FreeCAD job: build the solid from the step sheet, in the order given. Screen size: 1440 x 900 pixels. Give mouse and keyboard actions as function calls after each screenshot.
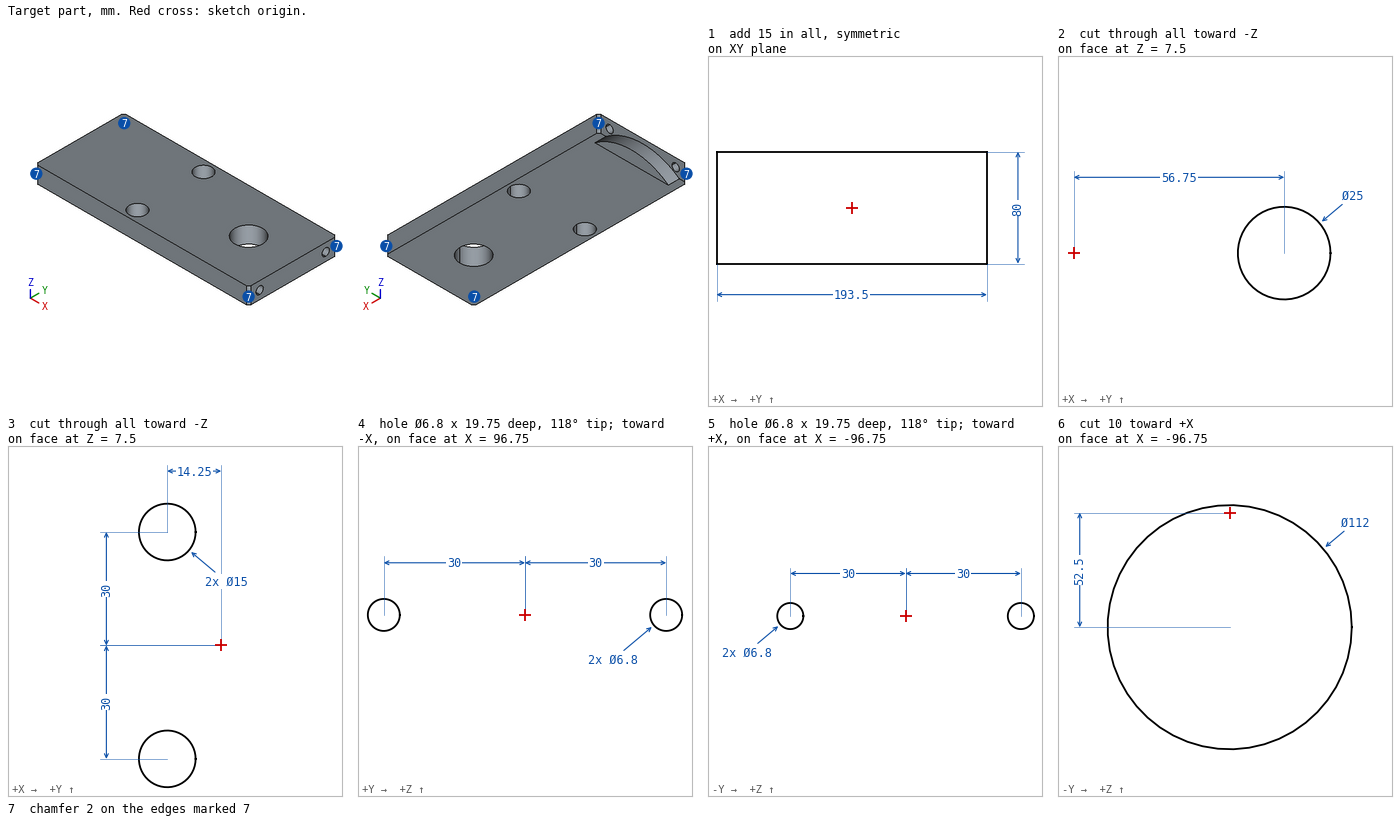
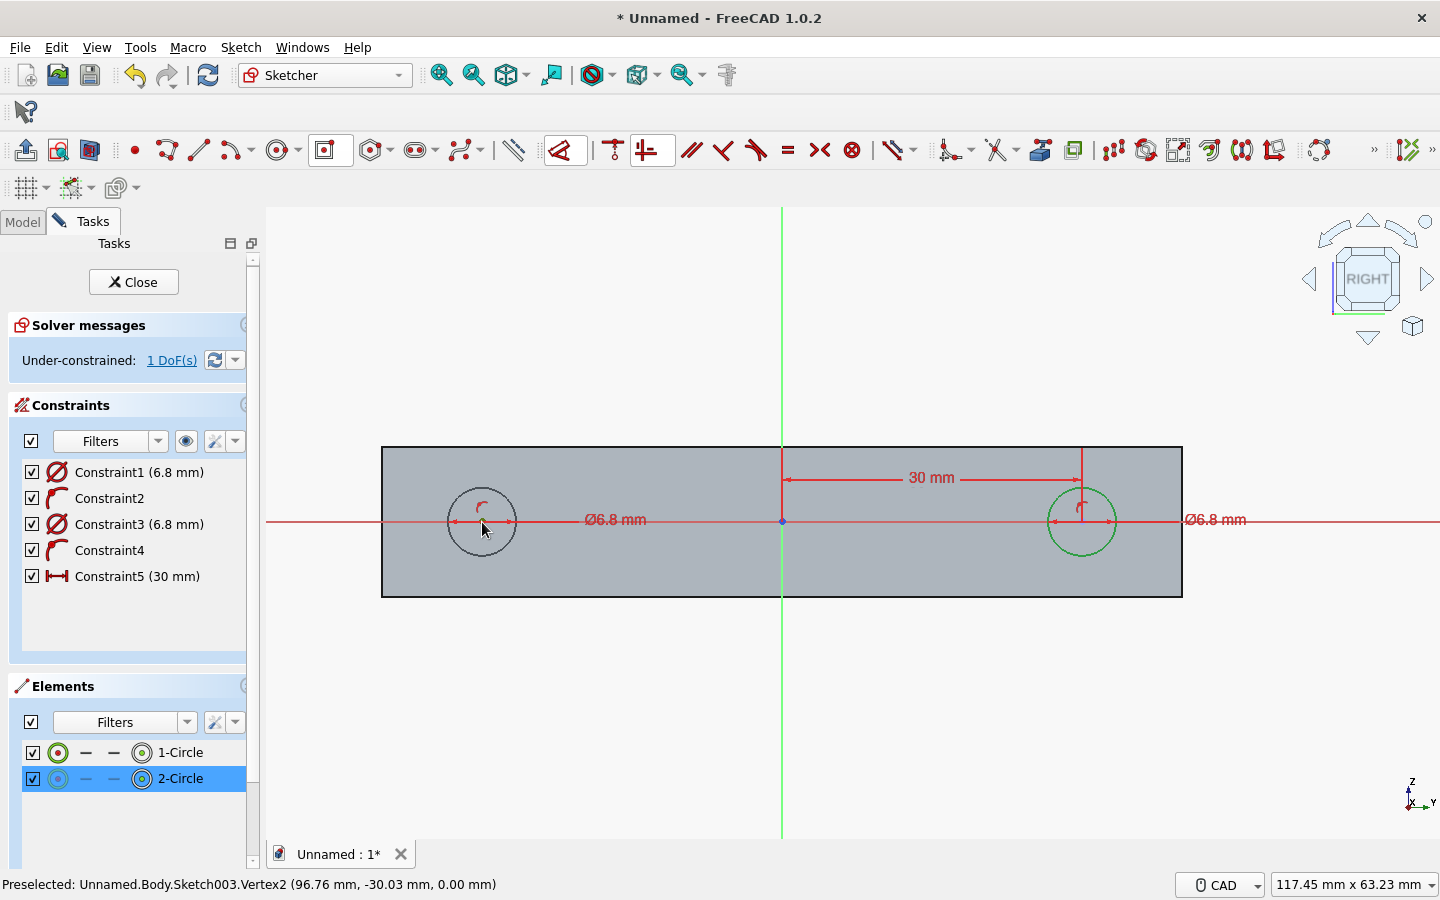
key(l)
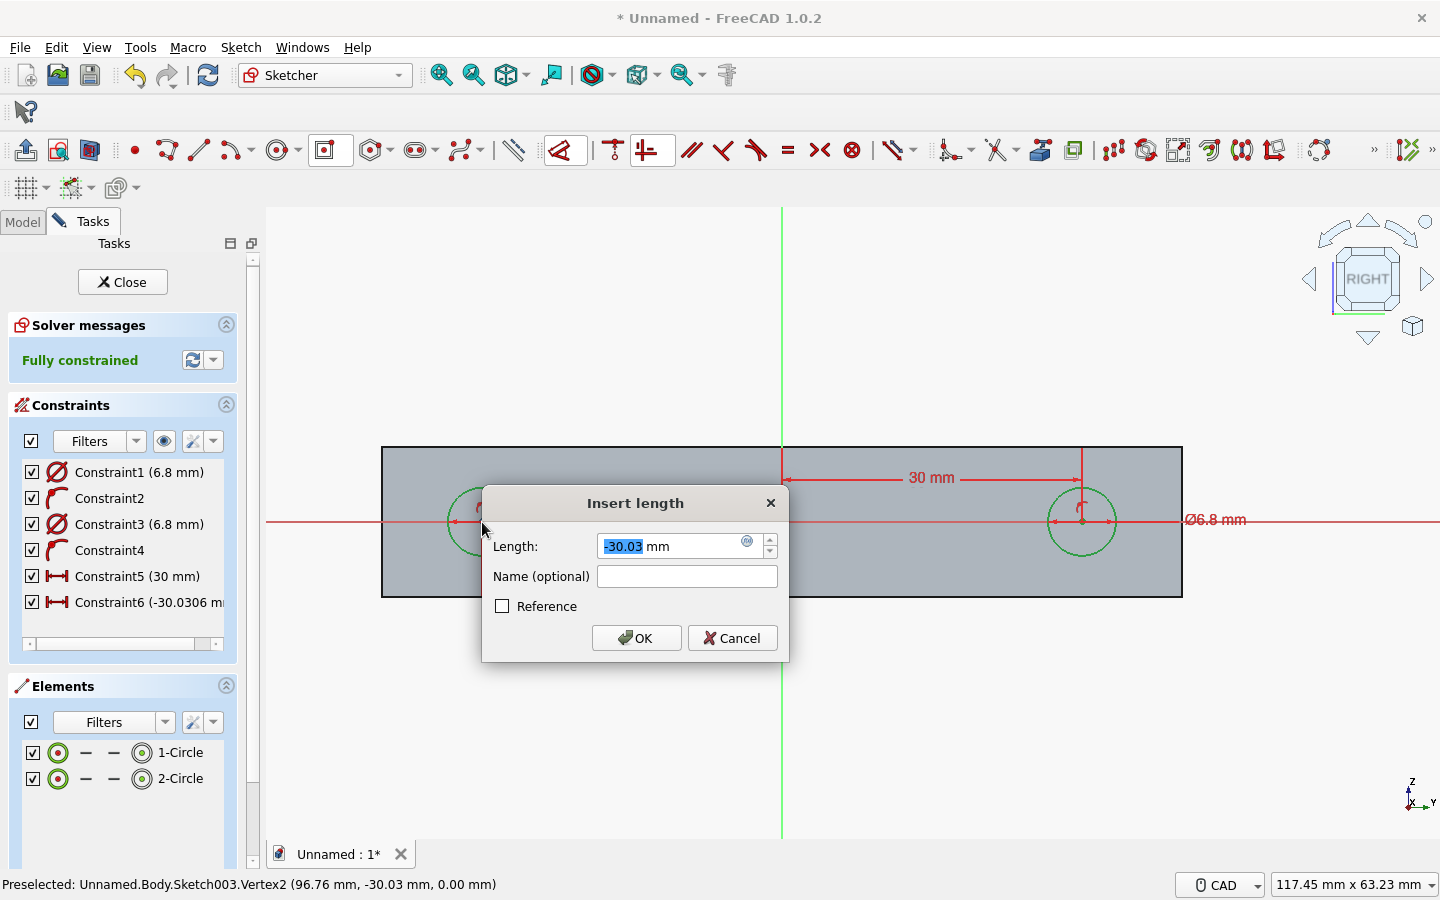
text(-30)
key(Return)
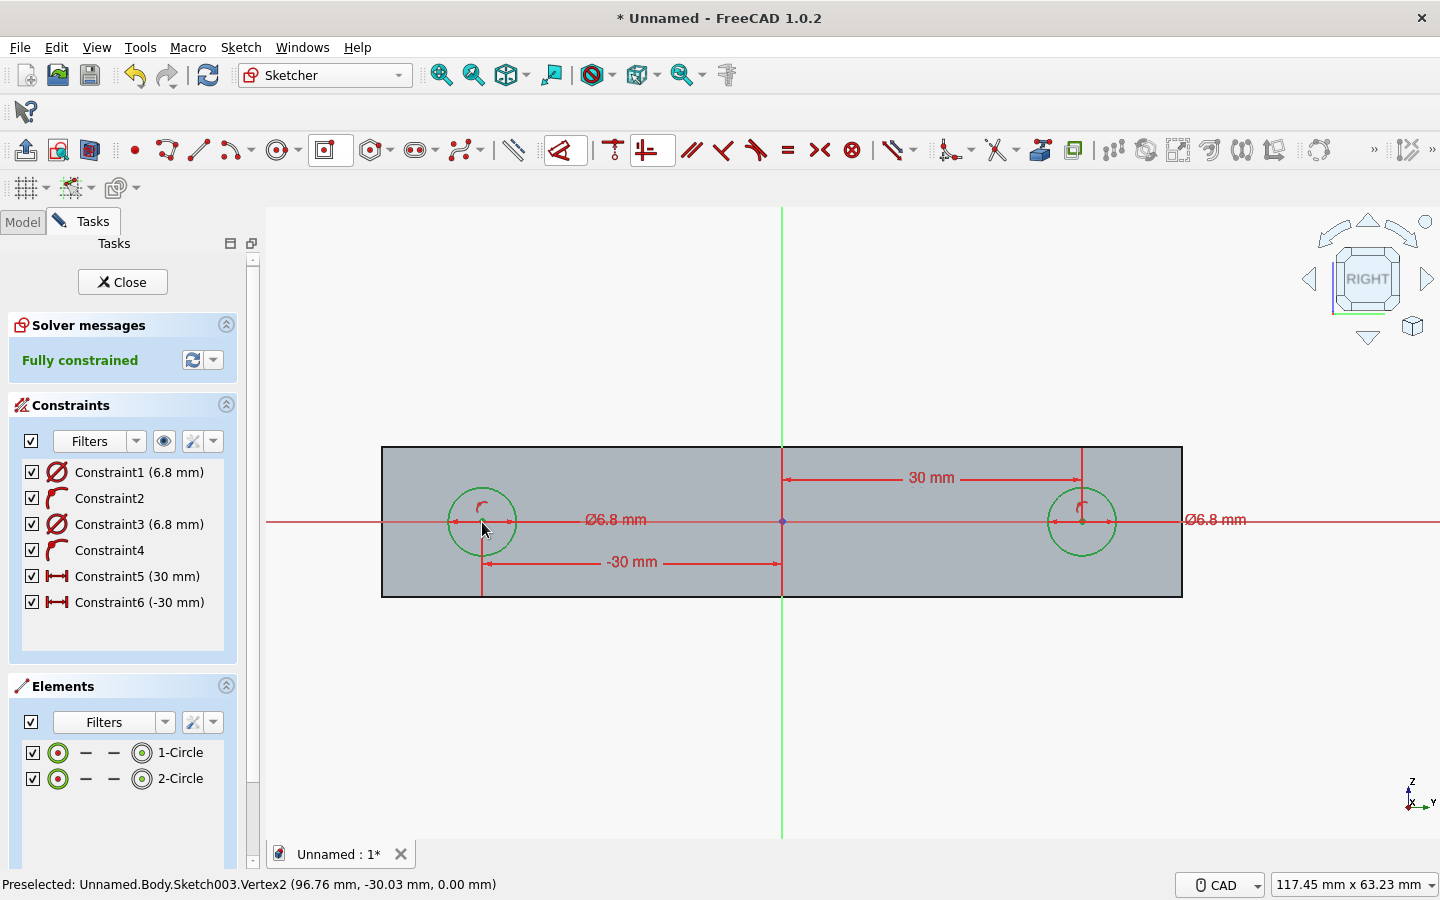
click(123, 282)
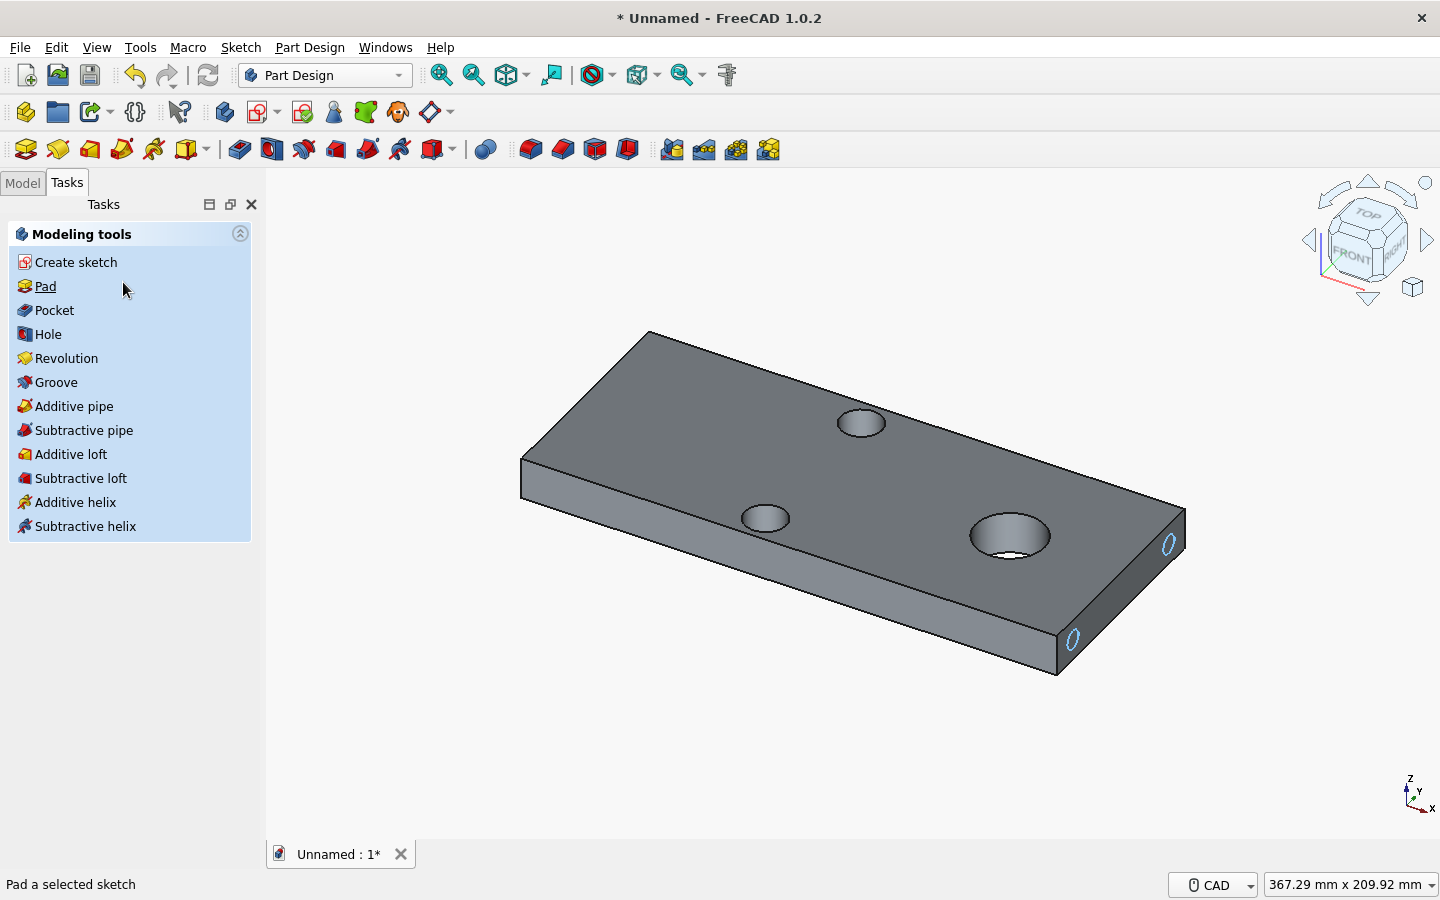
click(272, 150)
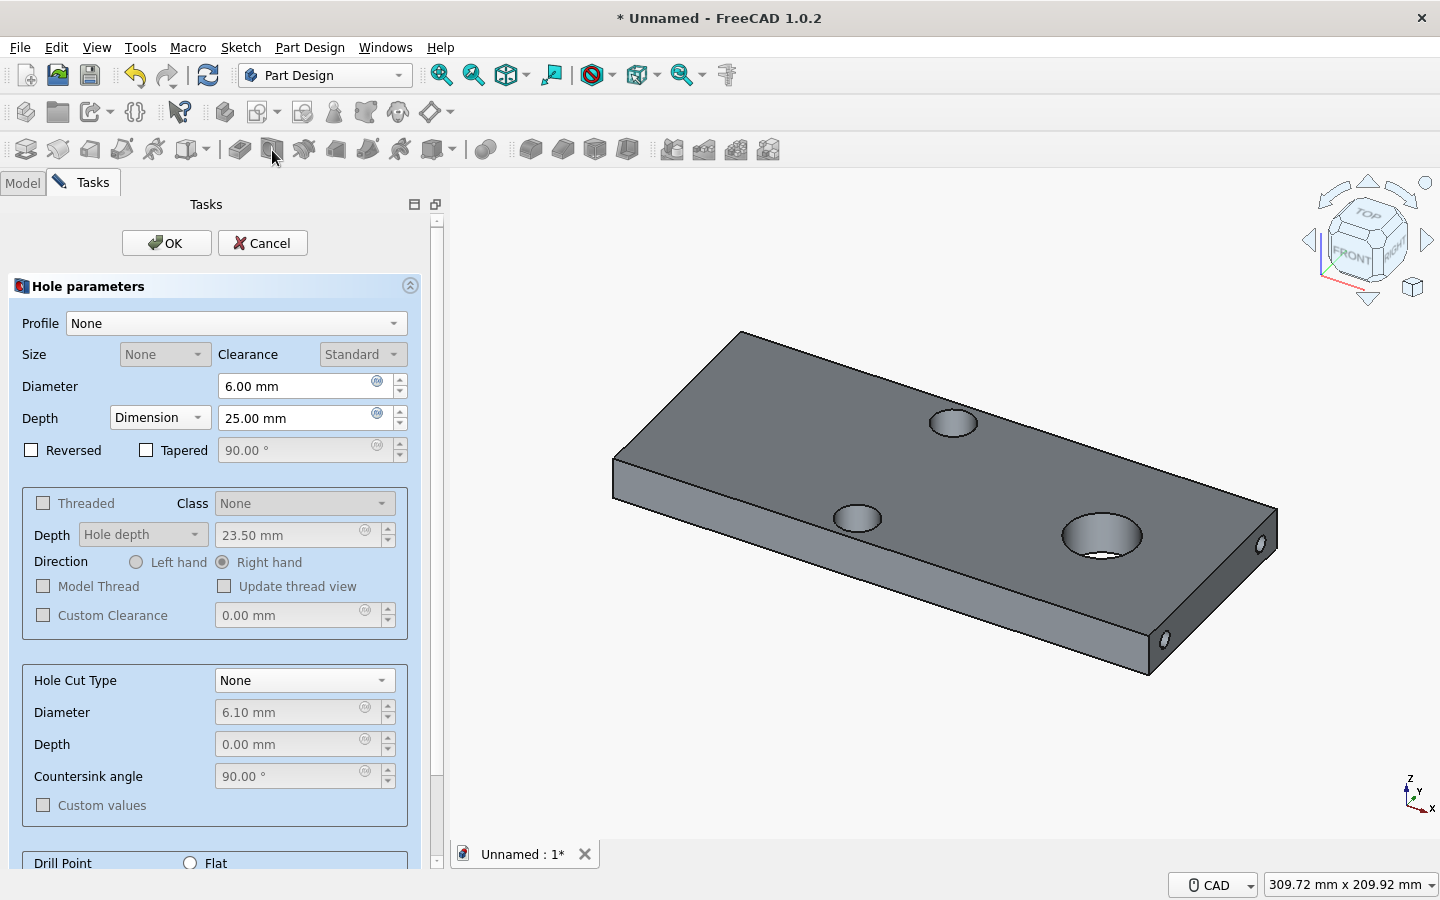
triple_click(305, 386)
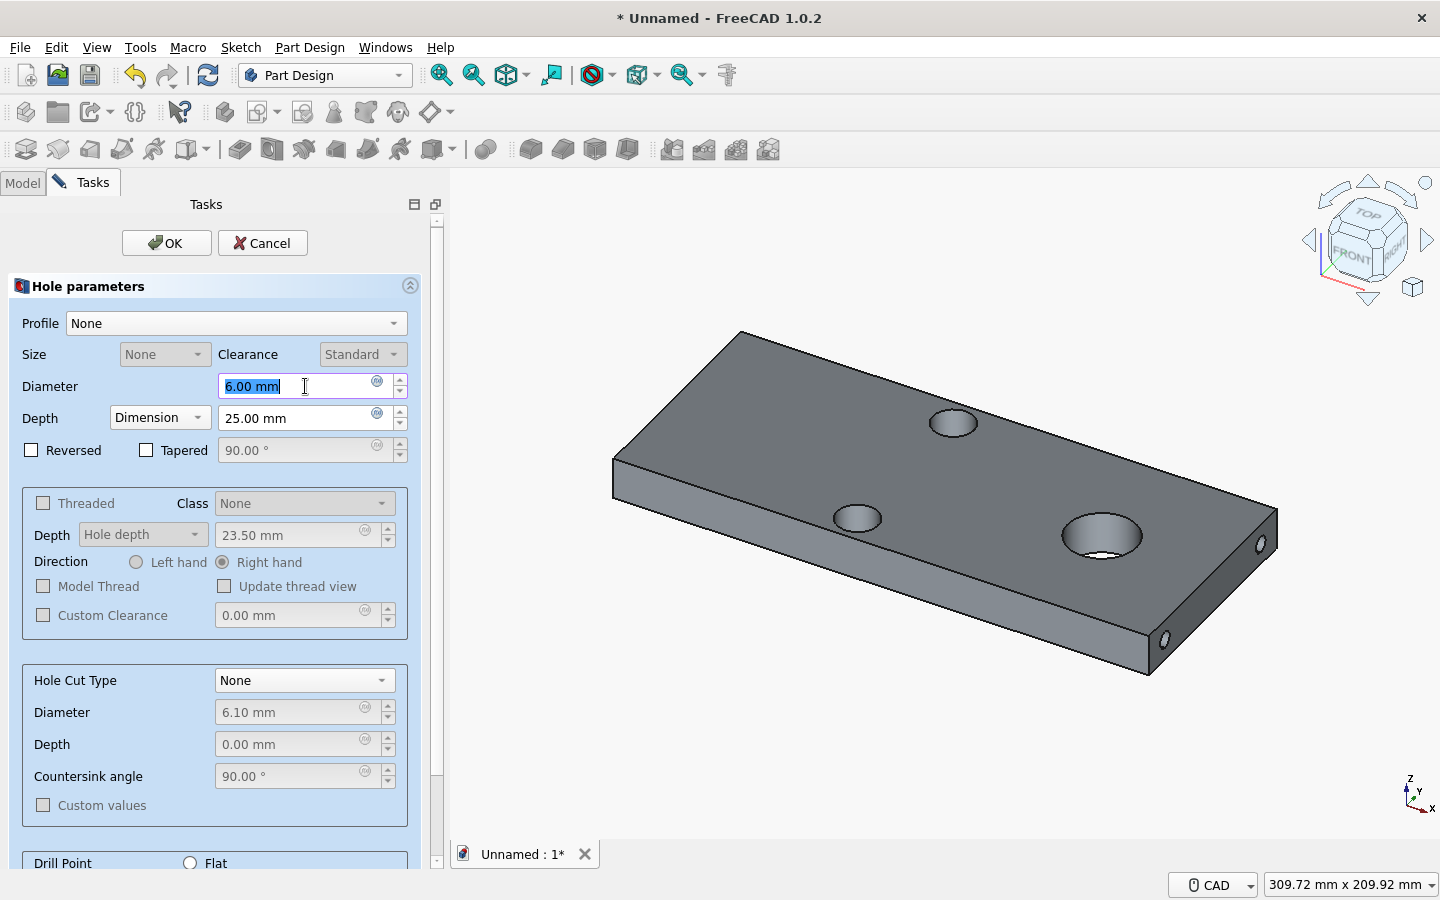
text(6.8)
key(Tab)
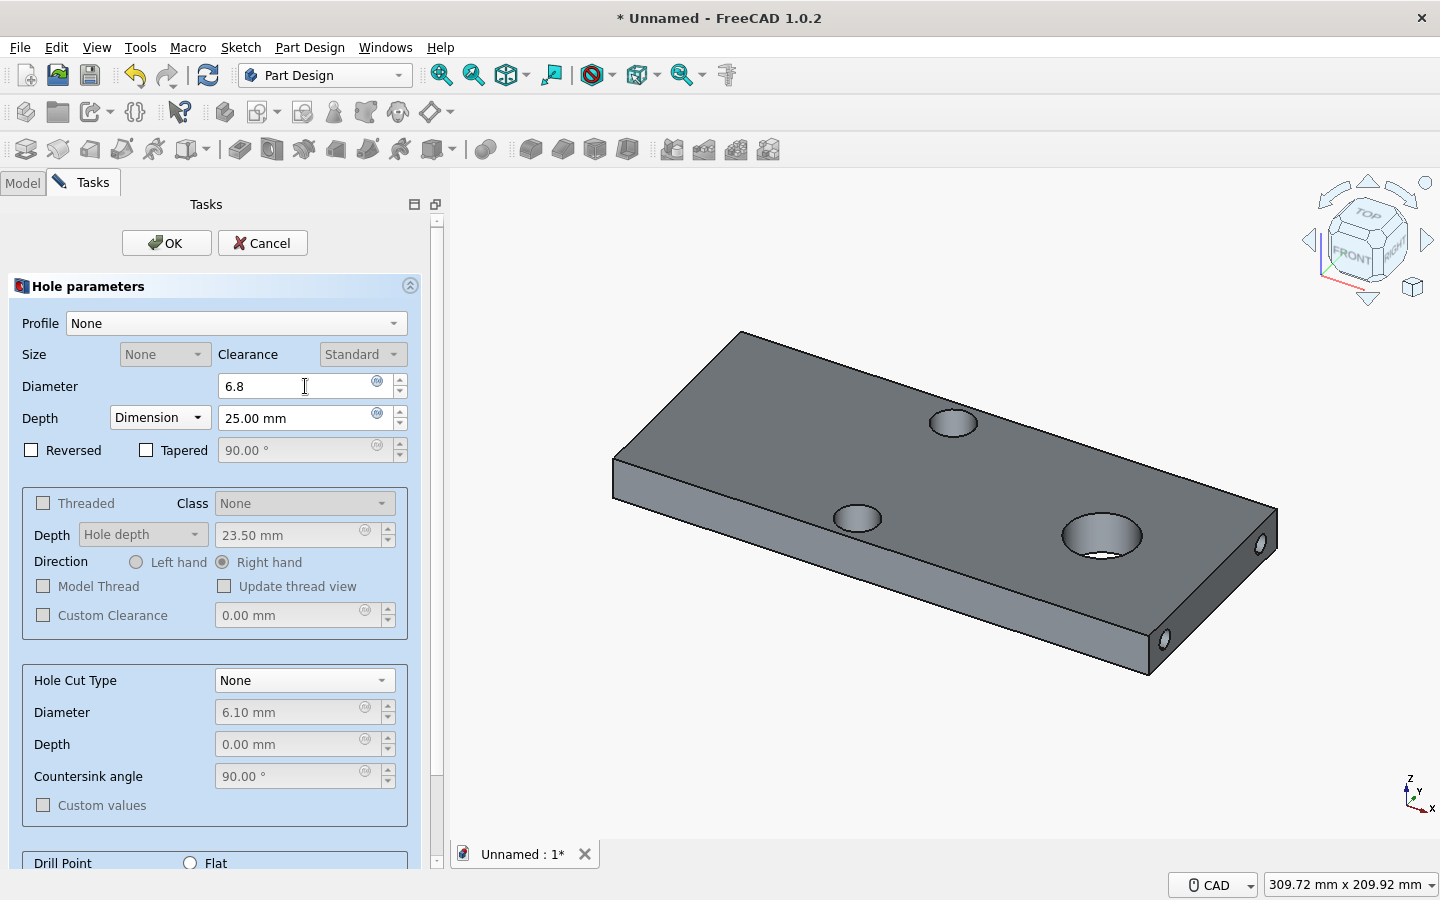
triple_click(305, 418)